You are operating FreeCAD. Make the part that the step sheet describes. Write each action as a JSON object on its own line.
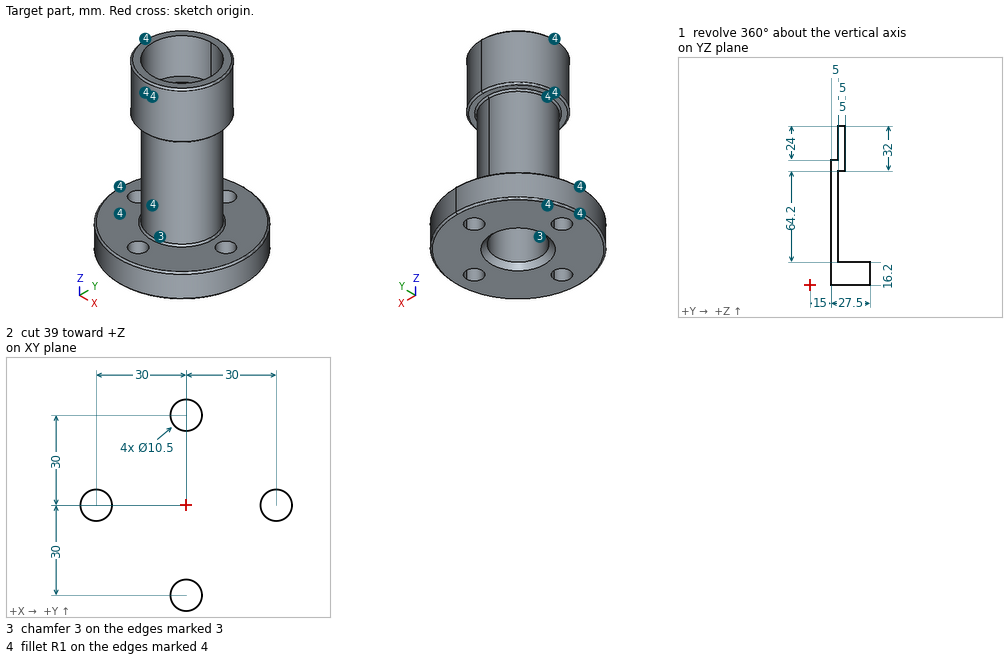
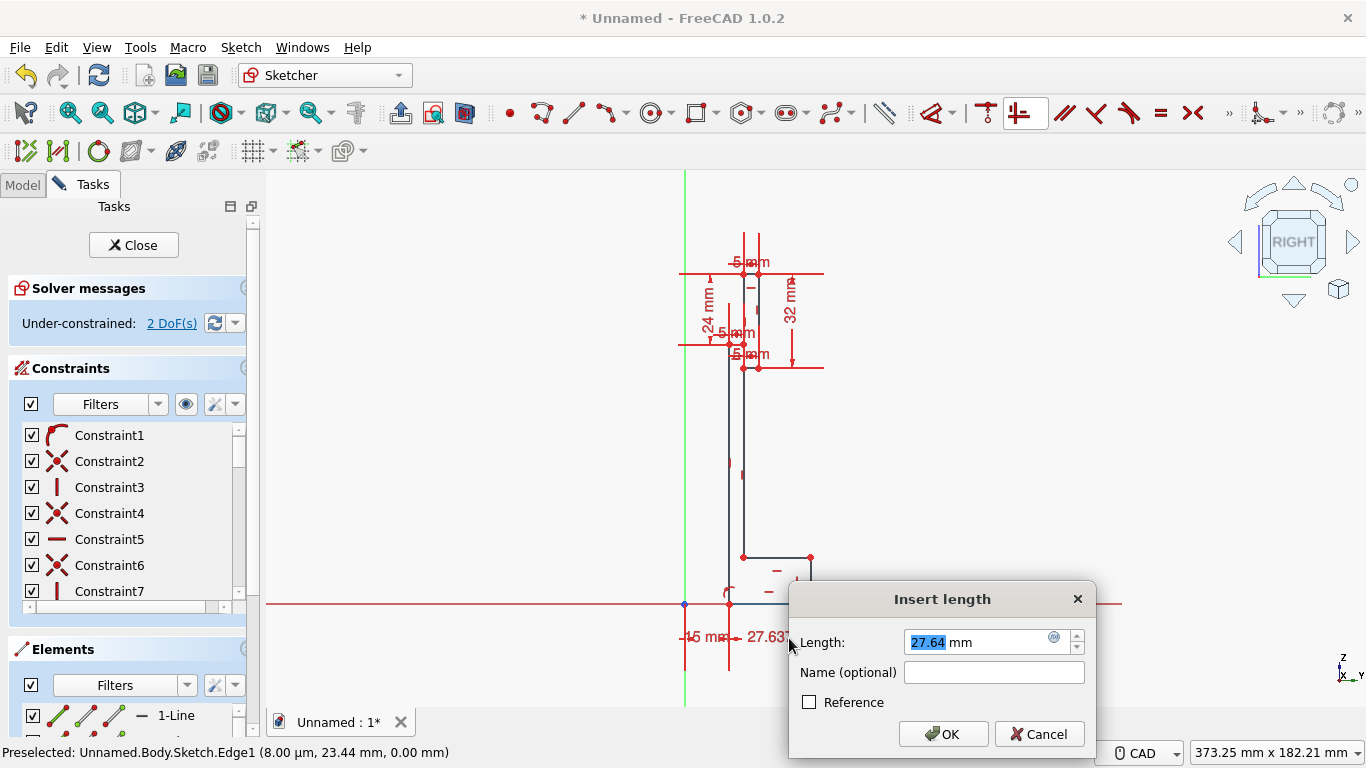
{"action": "type", "text": "27.5"}
{"action": "key", "text": "Return"}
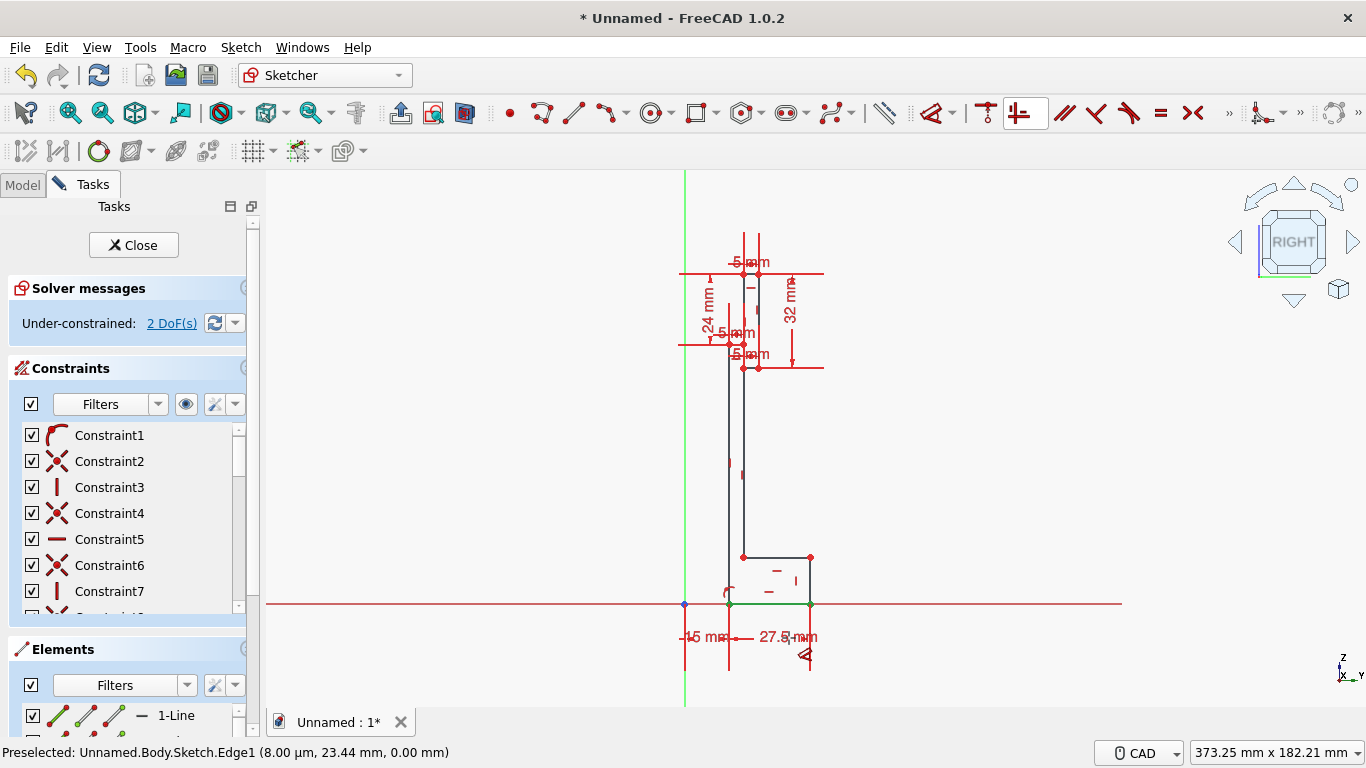
{"action": "left_click", "coordinate": [810, 590]}
{"action": "left_click", "coordinate": [844, 581]}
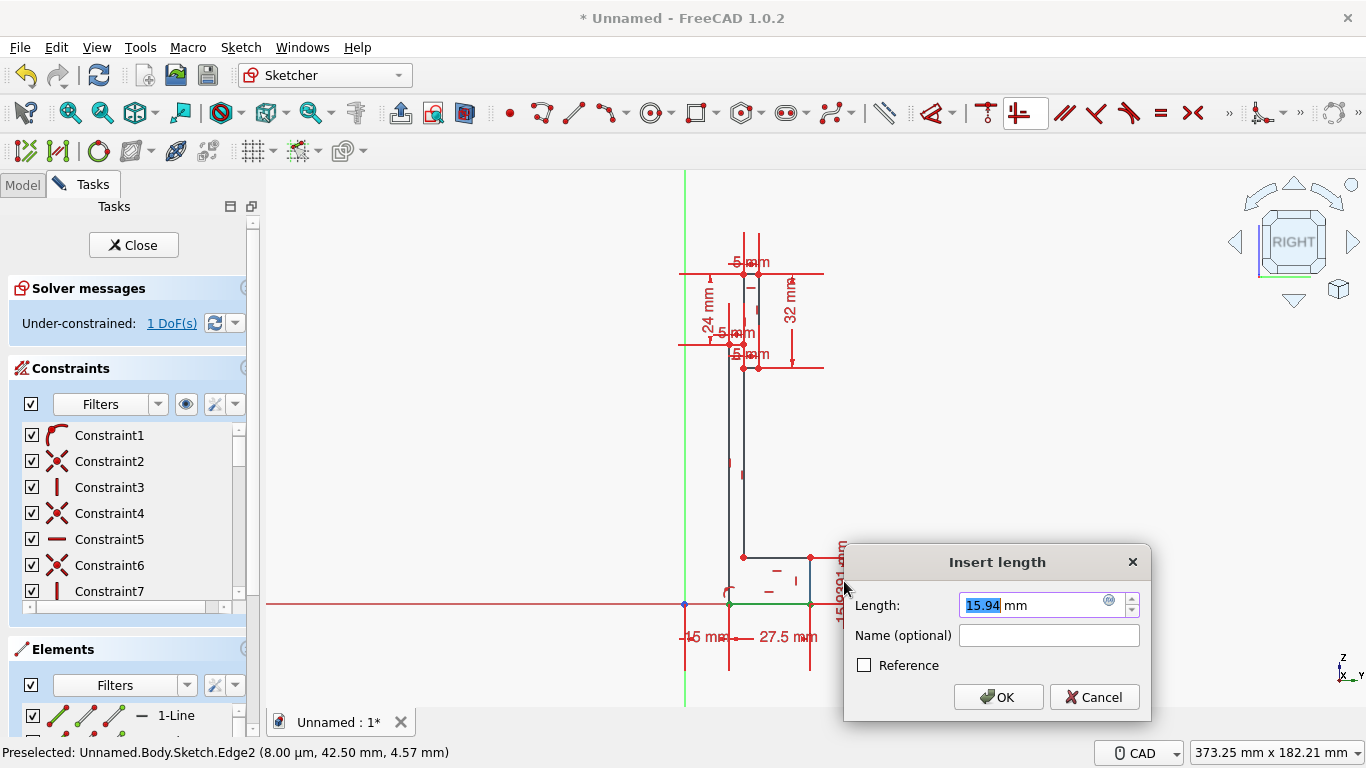
{"action": "type", "text": "16.2"}
{"action": "key", "text": "Return"}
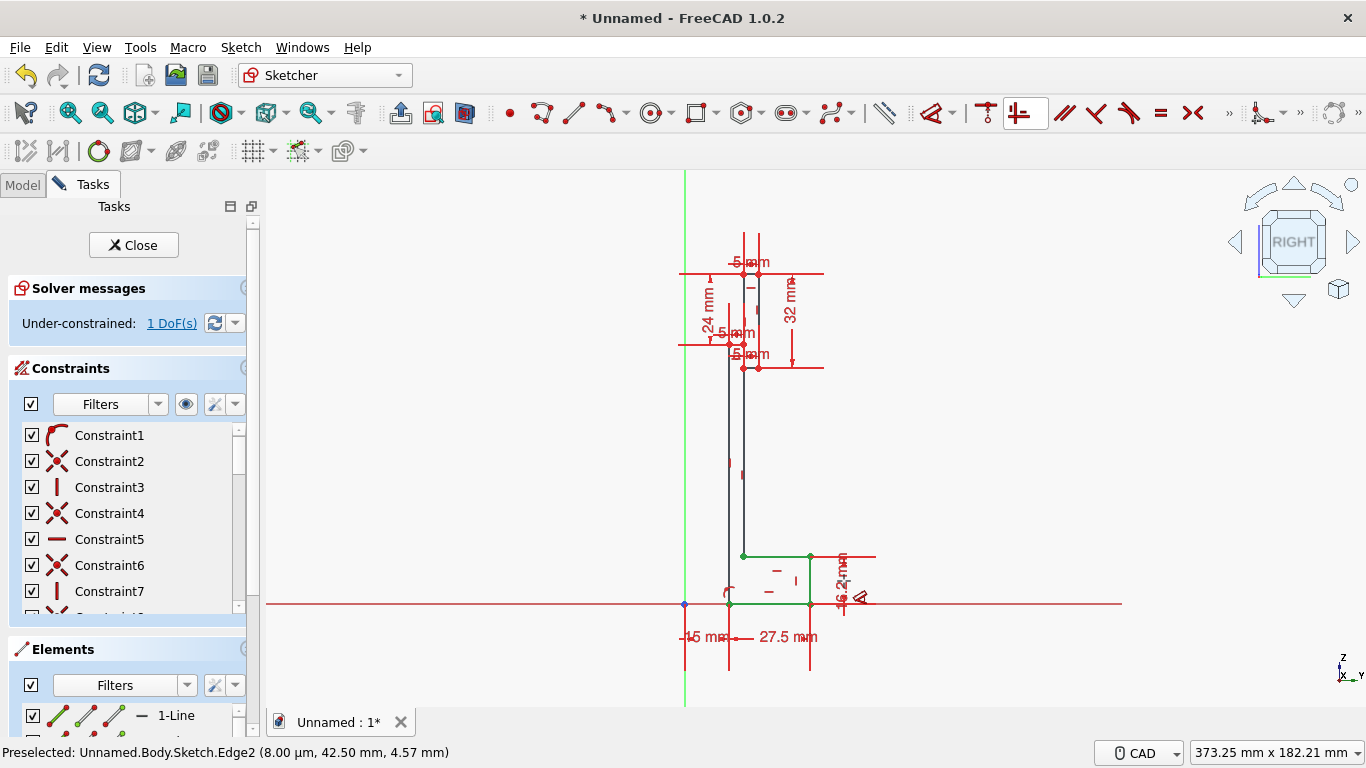
{"action": "left_click", "coordinate": [744, 500]}
{"action": "left_click", "coordinate": [710, 463]}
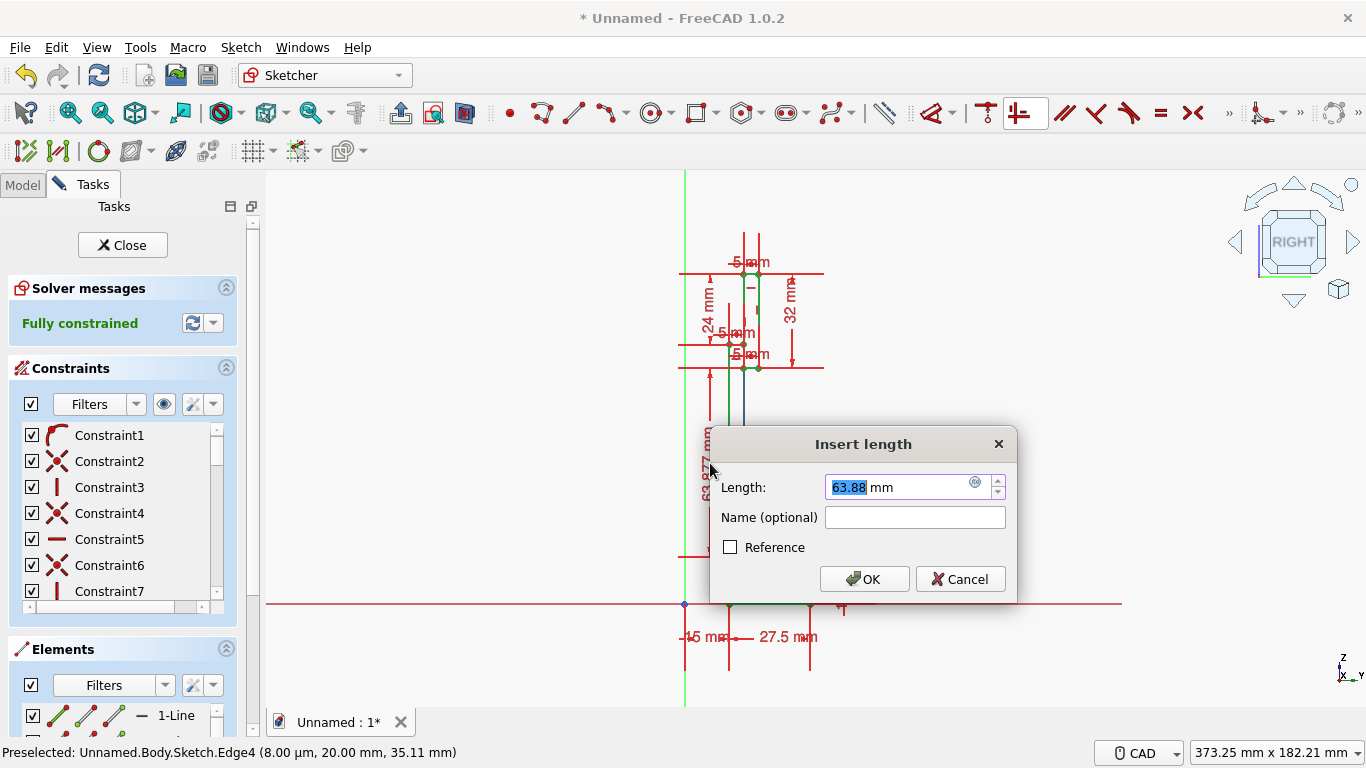
{"action": "type", "text": "64.2"}
{"action": "key", "text": "Return"}
{"action": "key", "text": "Escape"}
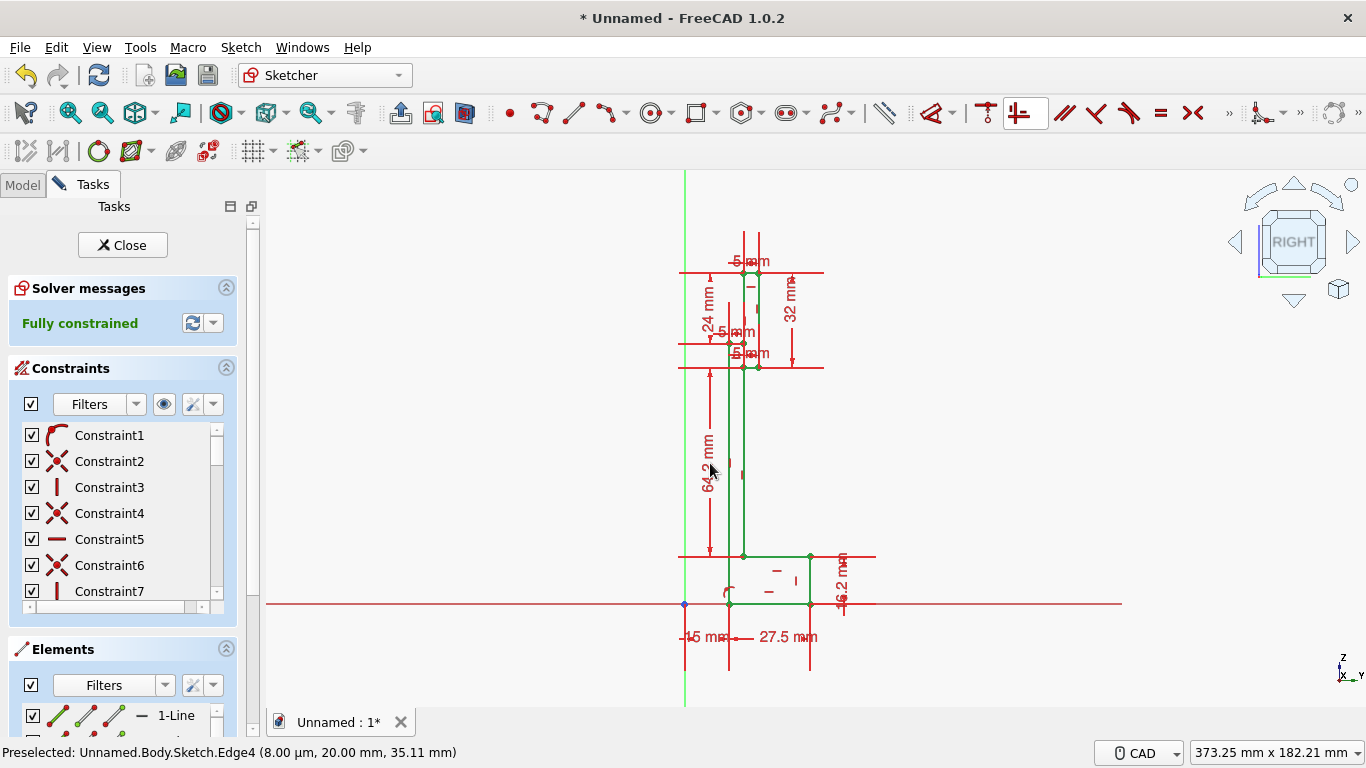
{"action": "left_click", "coordinate": [123, 245]}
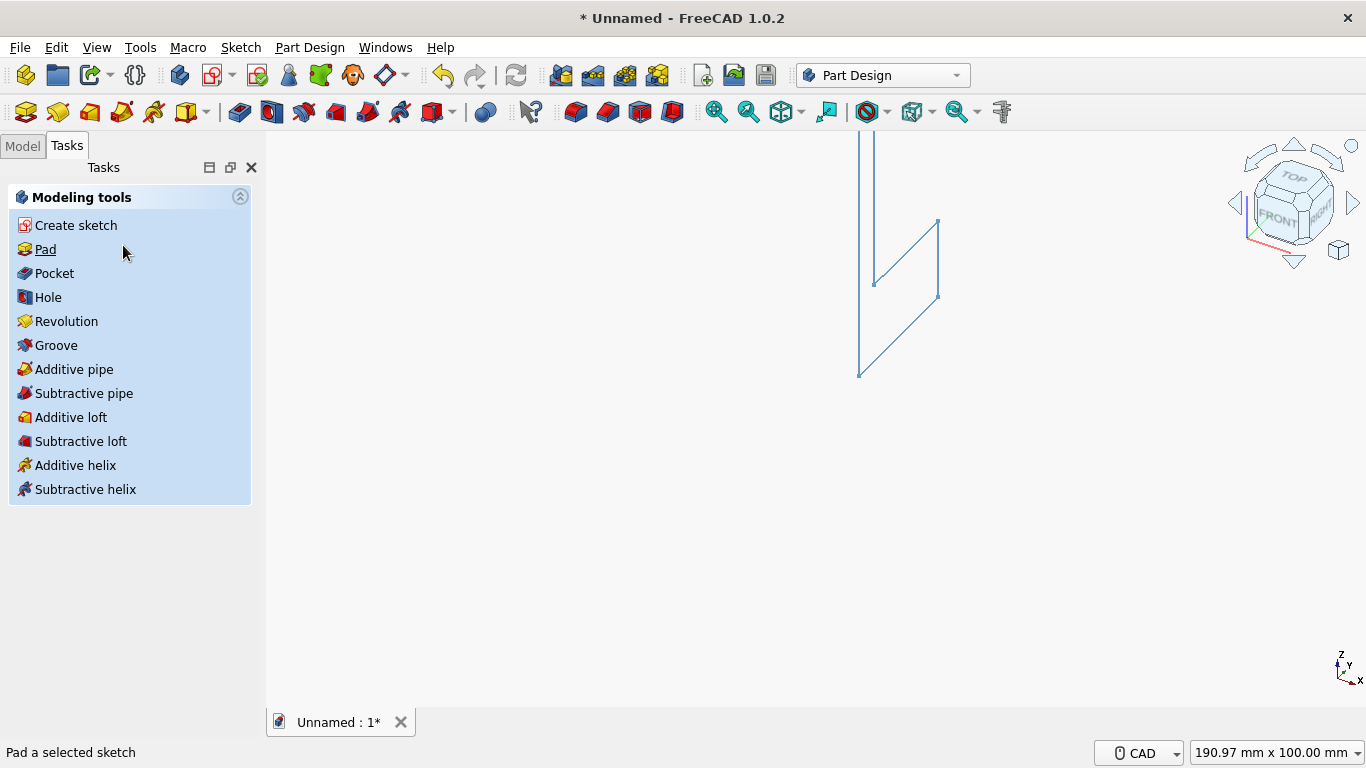
{"action": "left_click", "coordinate": [58, 112]}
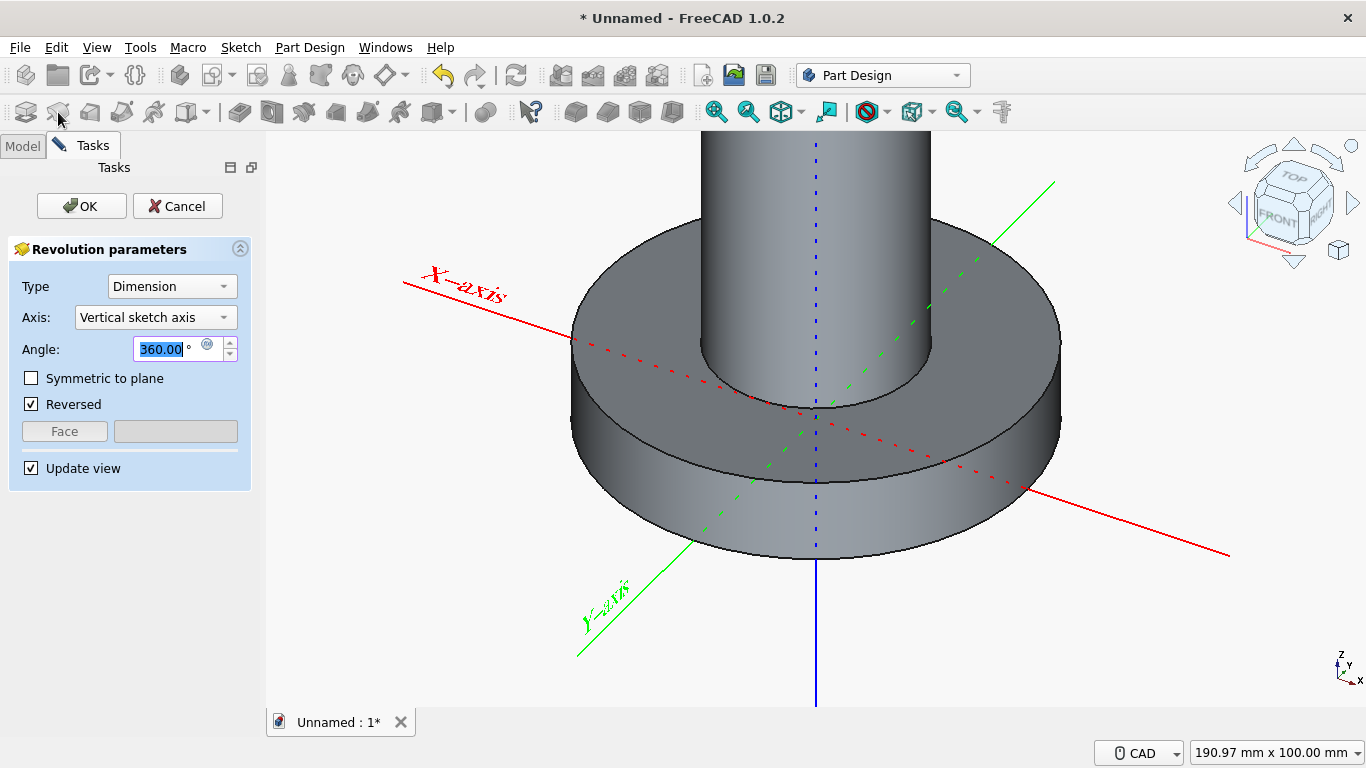
{"action": "left_click", "coordinate": [82, 206]}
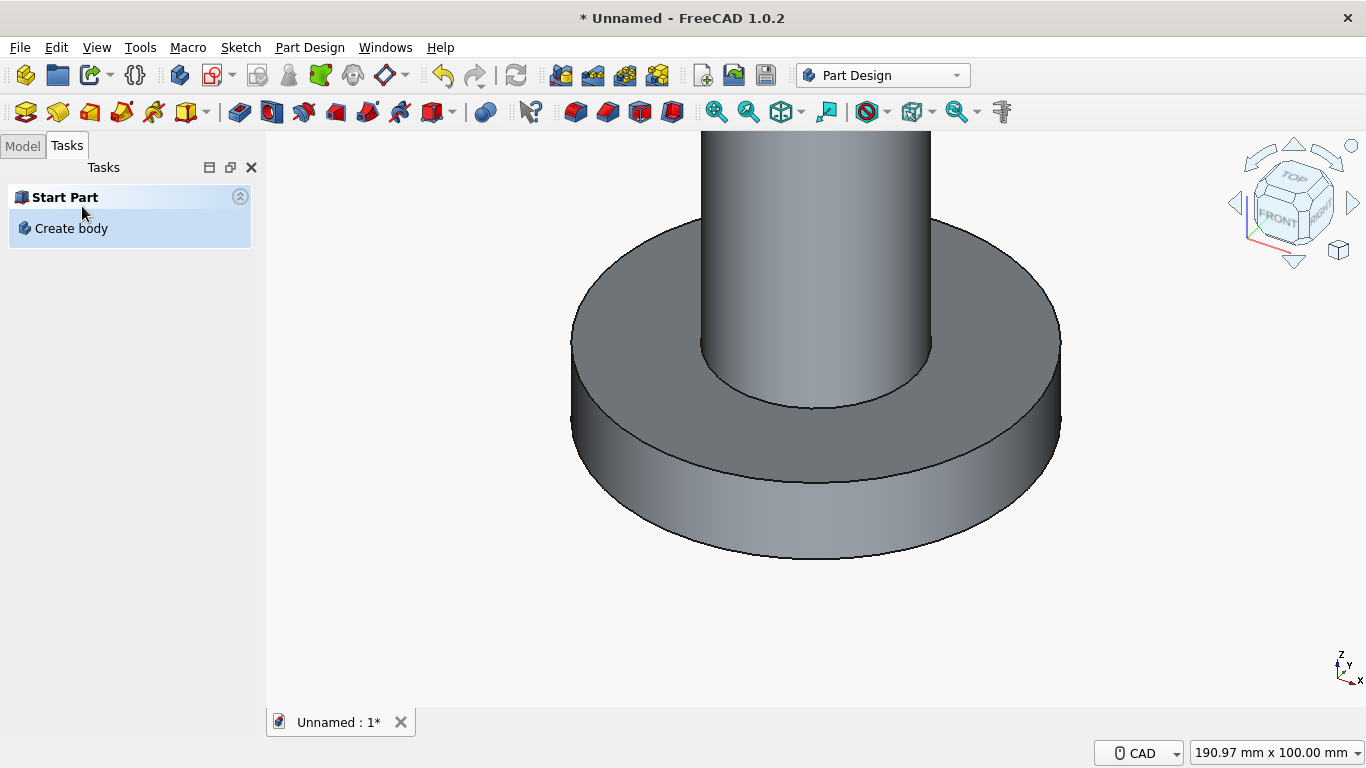
{"action": "left_click", "coordinate": [718, 112]}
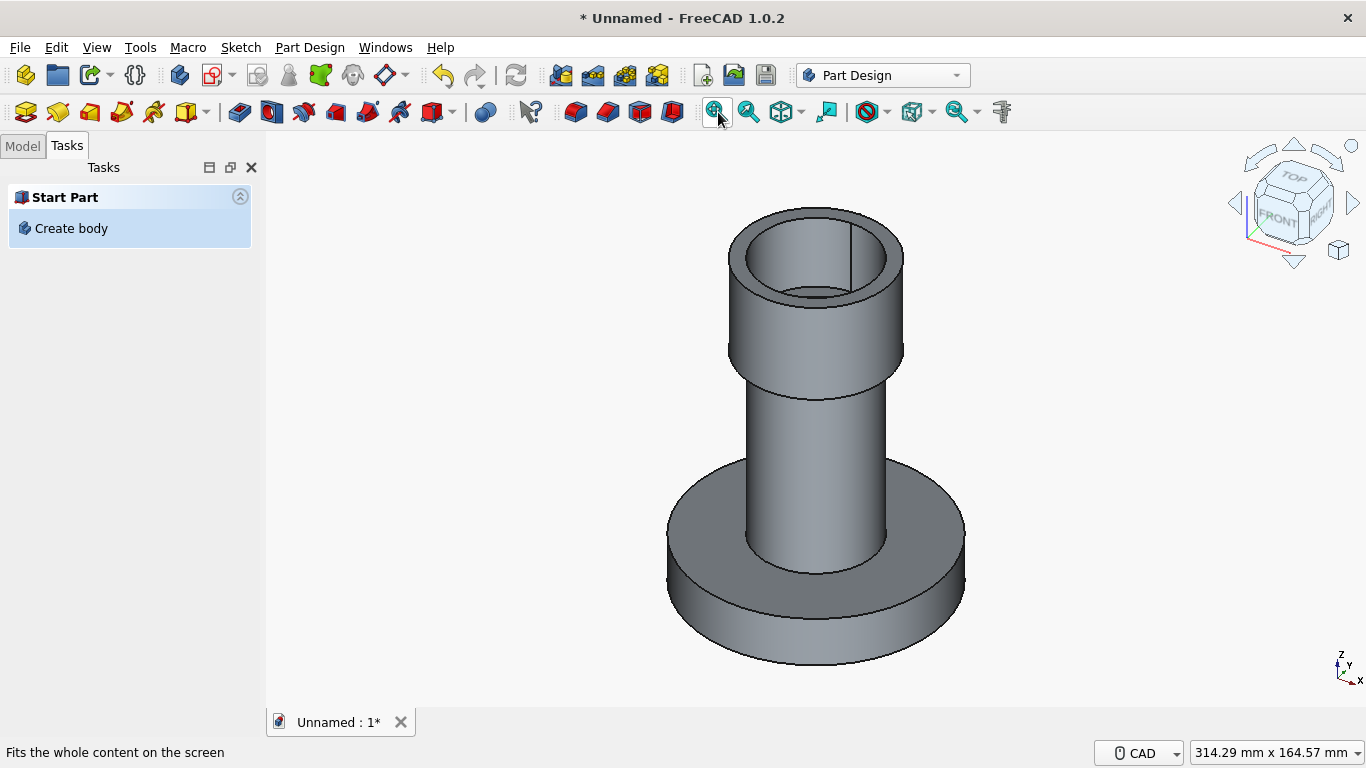
{"action": "left_click", "coordinate": [212, 76]}